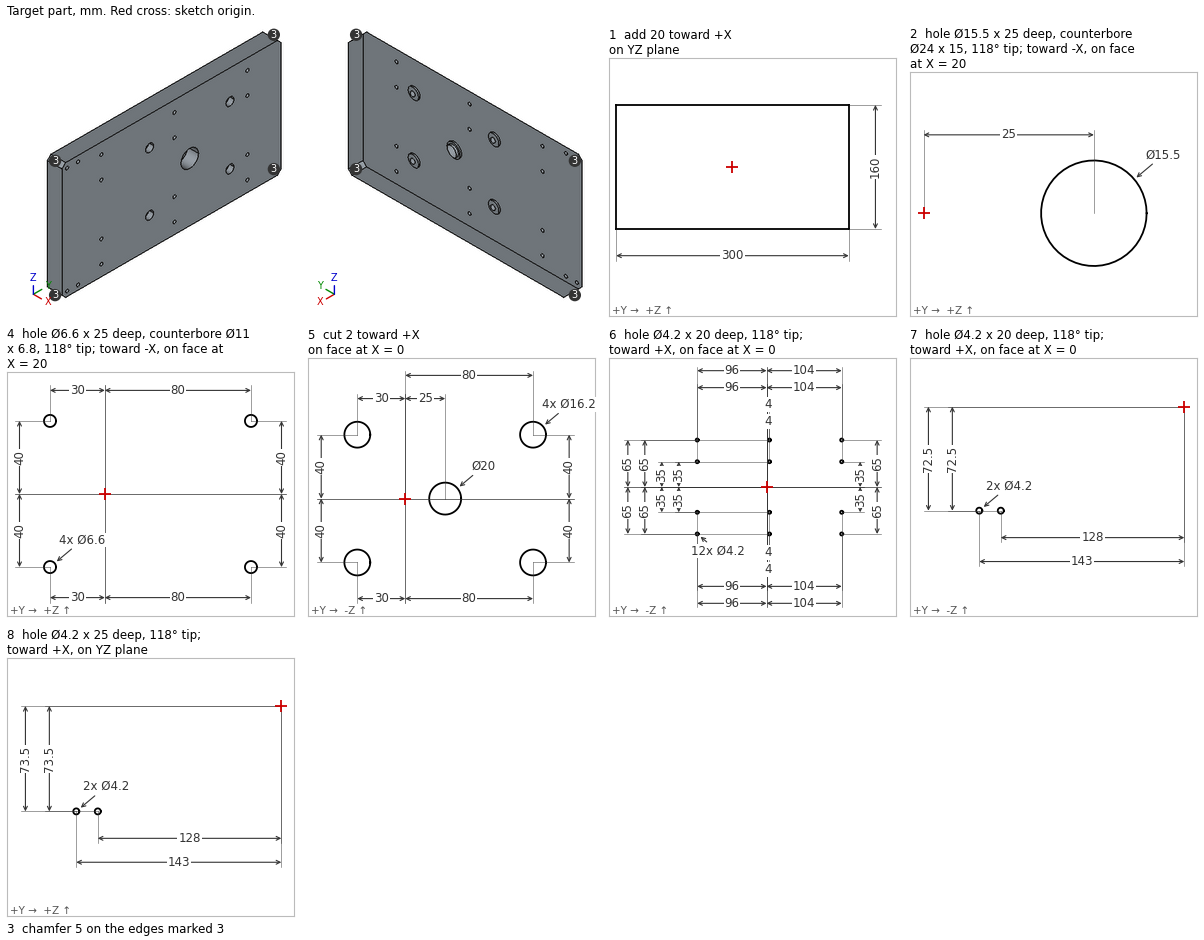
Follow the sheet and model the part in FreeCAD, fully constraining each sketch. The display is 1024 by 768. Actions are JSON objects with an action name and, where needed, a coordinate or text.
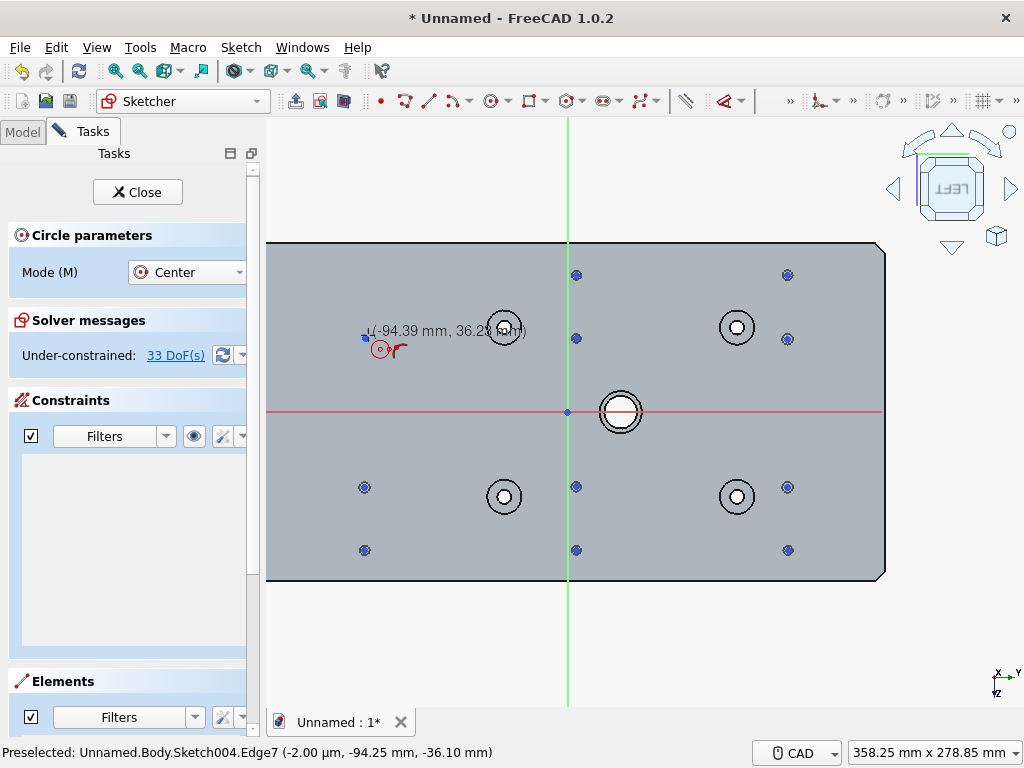
{"action": "scroll", "coordinate": [365, 275], "scroll_direction": "up", "scroll_amount": 9}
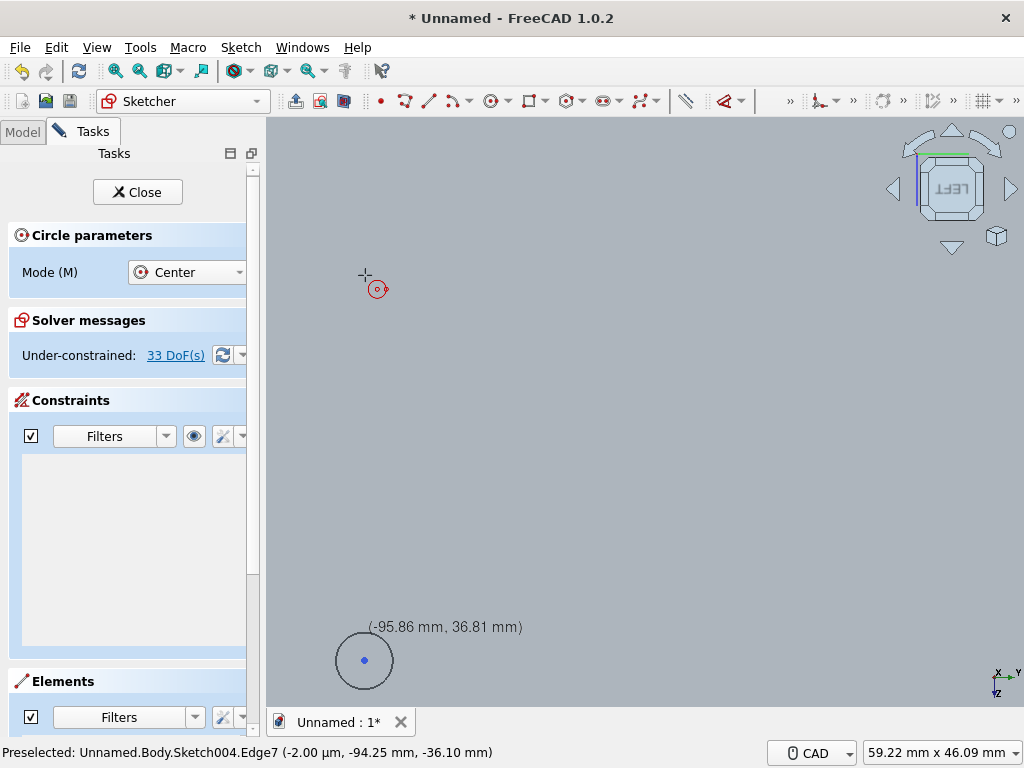
{"action": "scroll", "coordinate": [365, 275], "scroll_direction": "down", "scroll_amount": 9}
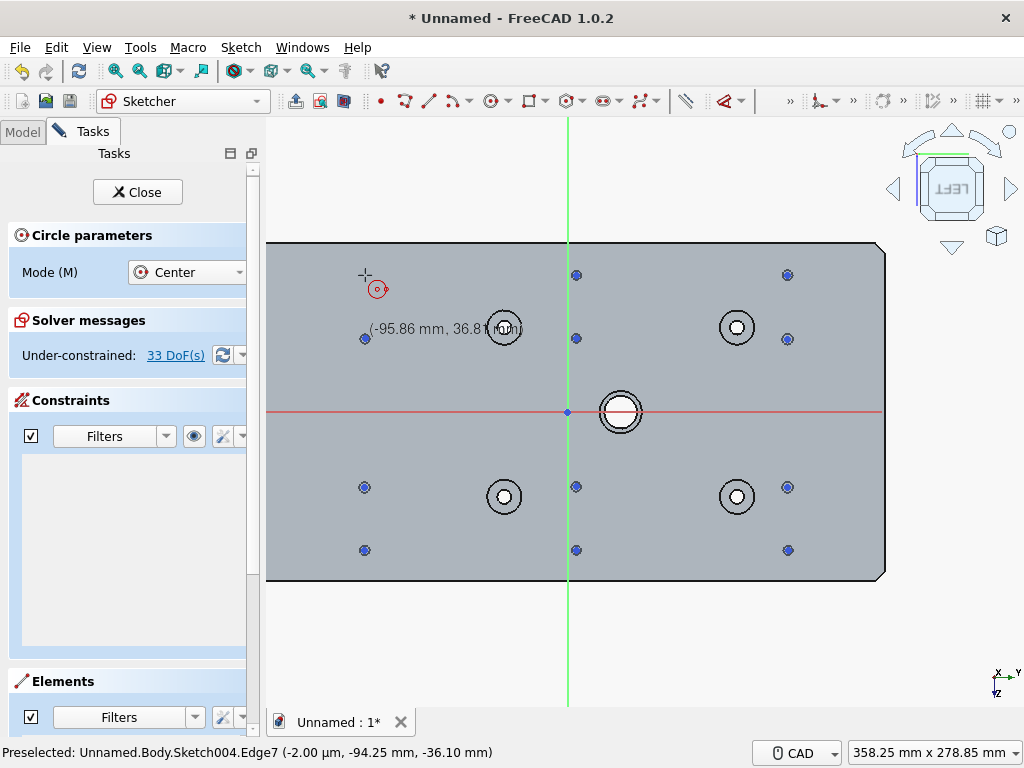
{"action": "left_click", "coordinate": [365, 275]}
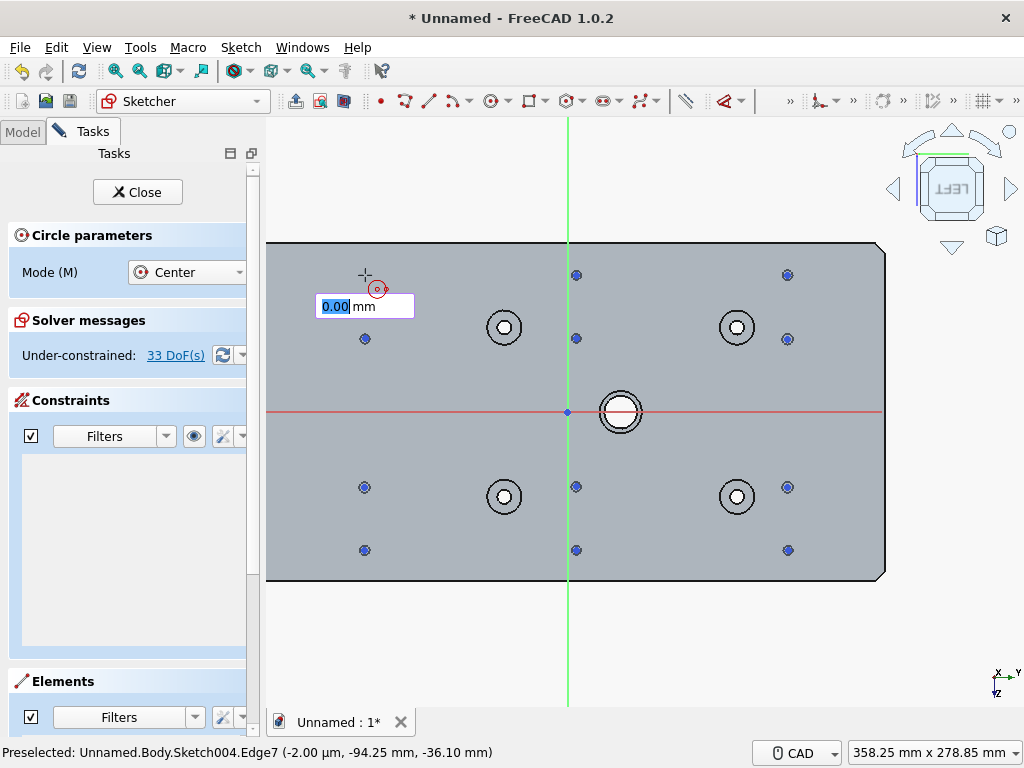
{"action": "scroll", "coordinate": [368, 272], "scroll_direction": "up", "scroll_amount": 7}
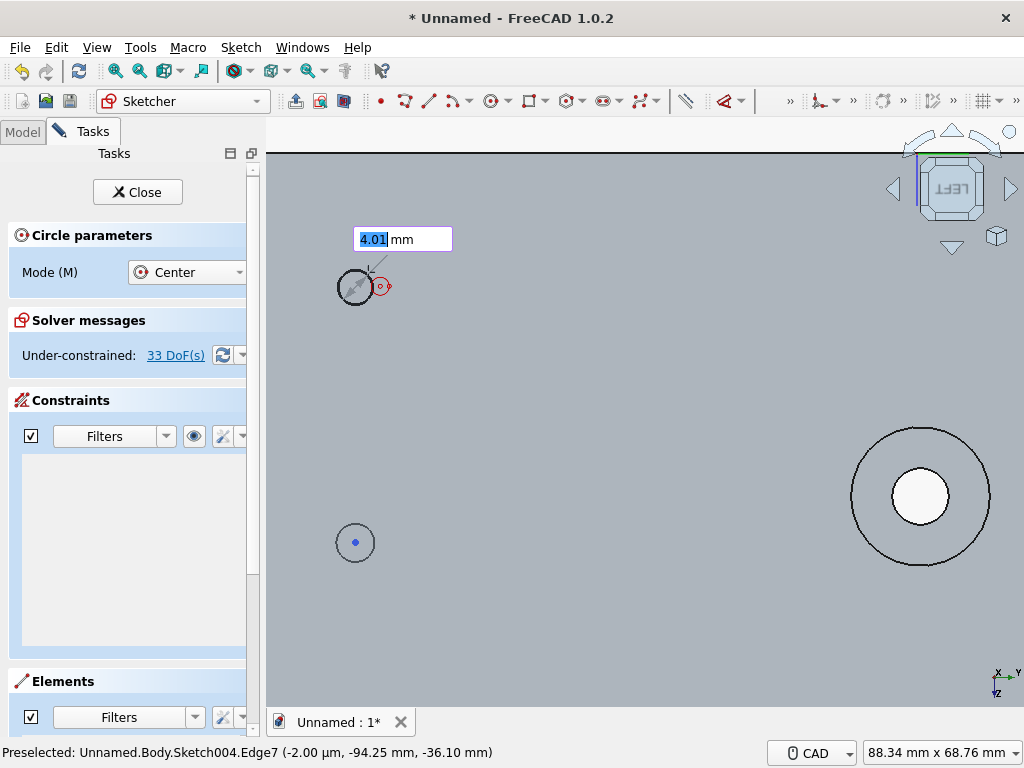
{"action": "left_click", "coordinate": [367, 269]}
{"action": "key", "text": "Escape"}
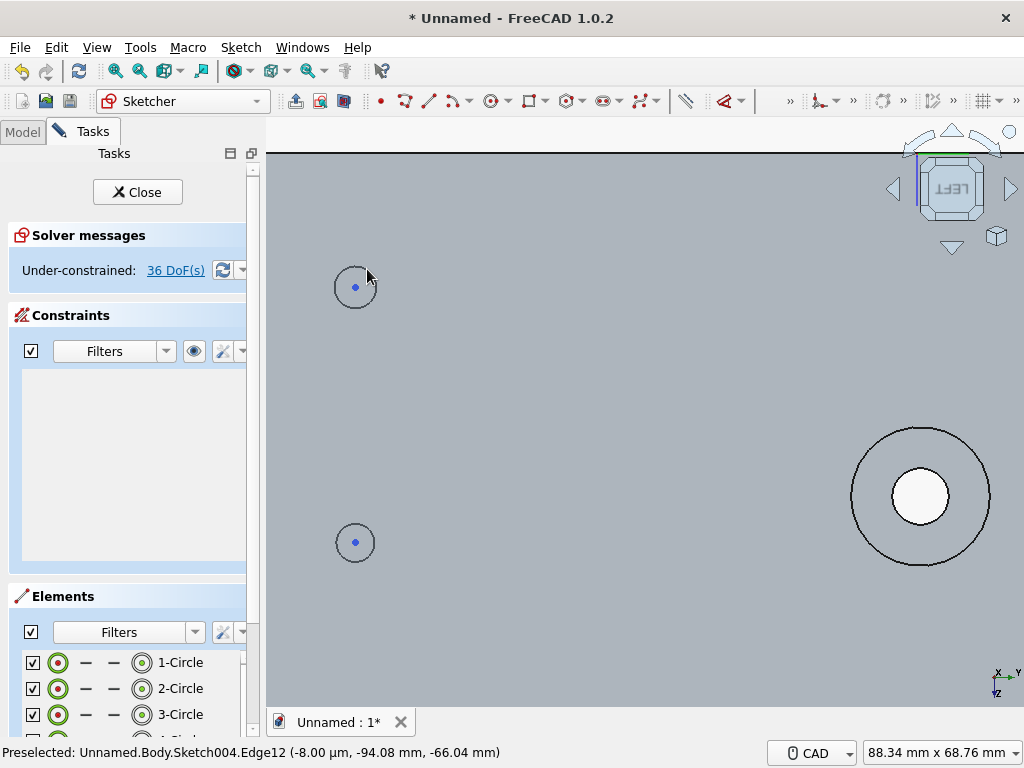
{"action": "scroll", "coordinate": [368, 272], "scroll_direction": "down", "scroll_amount": 7}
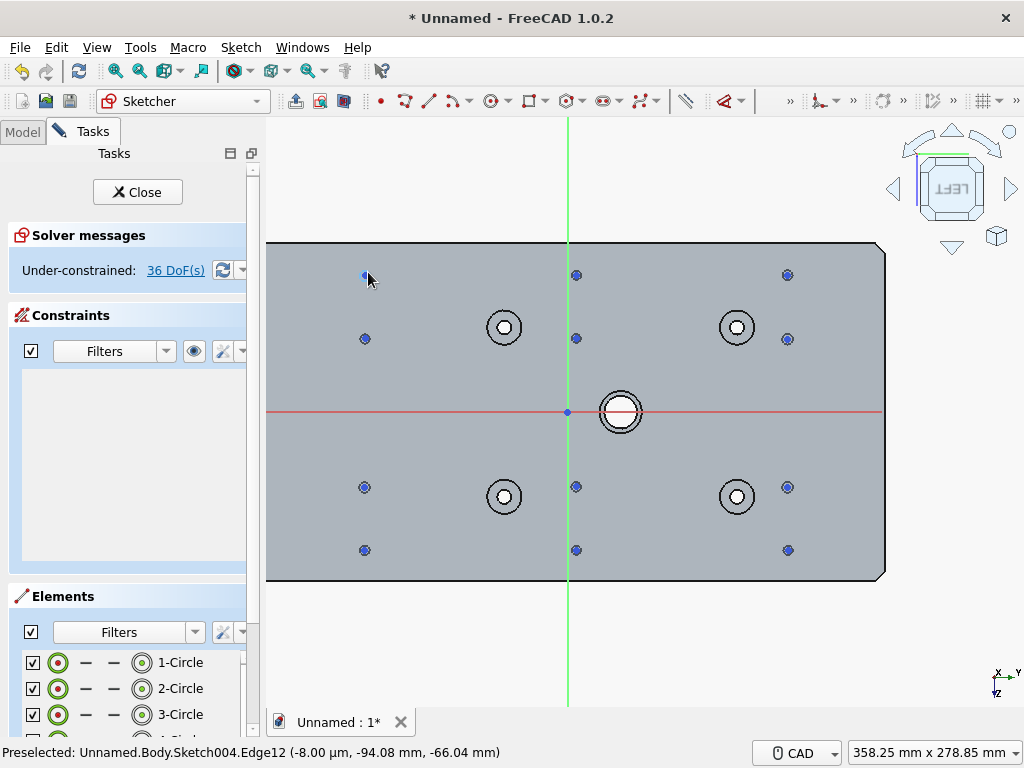
{"action": "scroll", "coordinate": [368, 547], "scroll_direction": "up", "scroll_amount": 6}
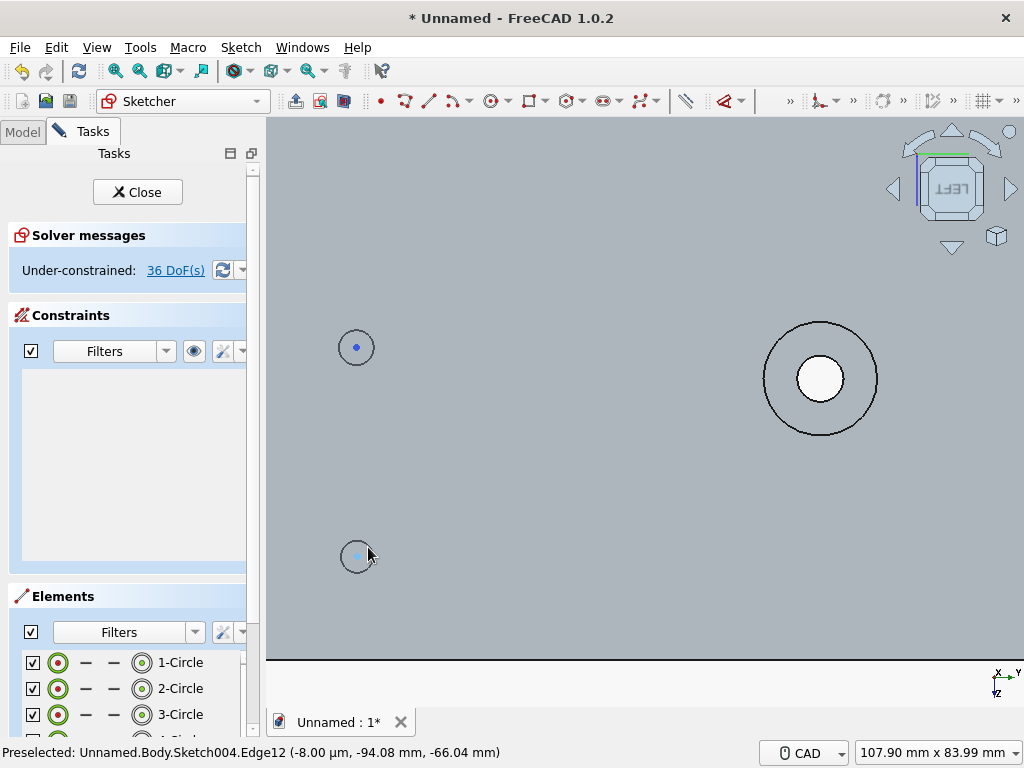
{"action": "left_click", "coordinate": [368, 545]}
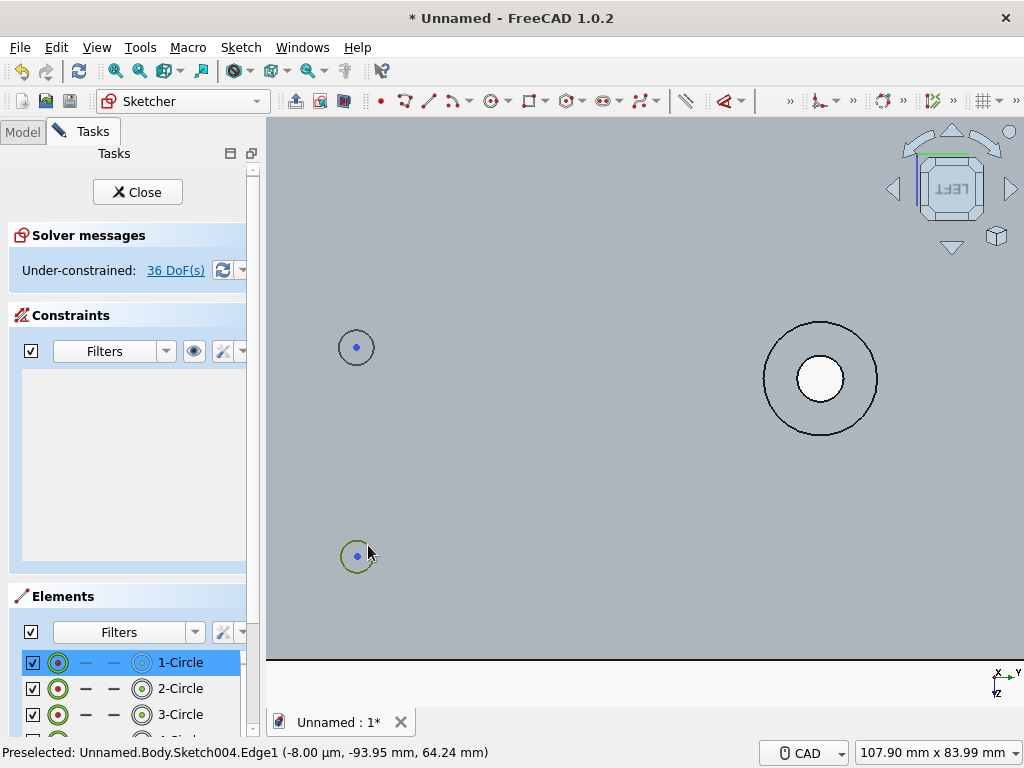
{"action": "left_click", "coordinate": [369, 335]}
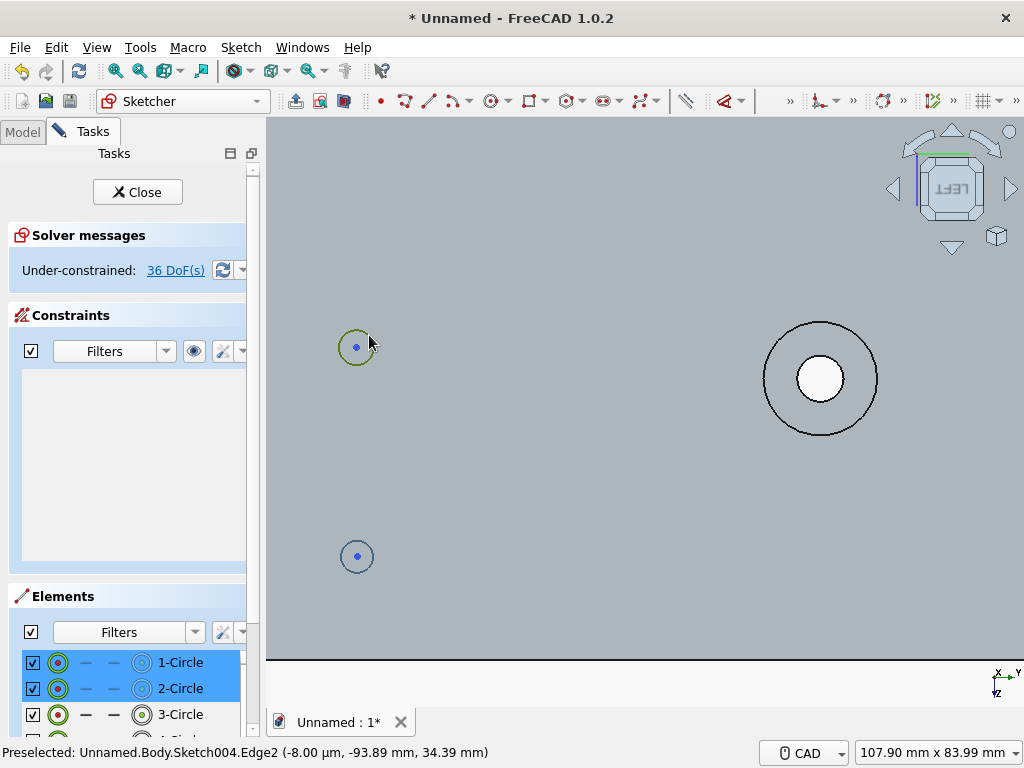
{"action": "scroll", "coordinate": [368, 547], "scroll_direction": "down", "scroll_amount": 6}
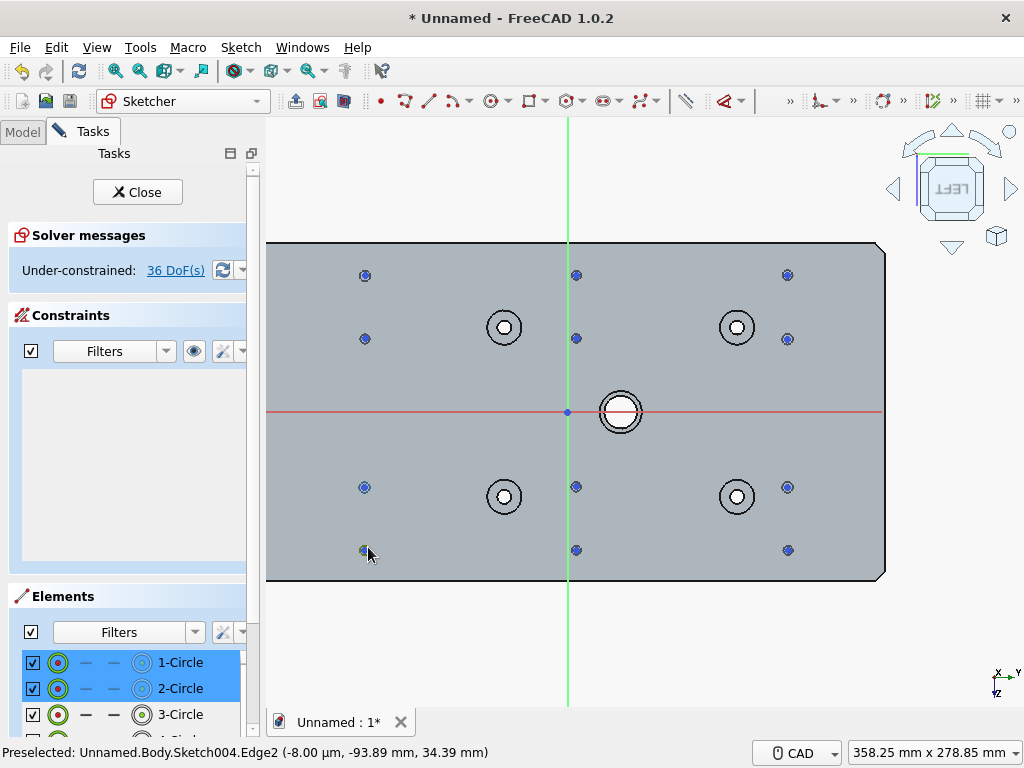
{"action": "scroll", "coordinate": [580, 547], "scroll_direction": "up", "scroll_amount": 6}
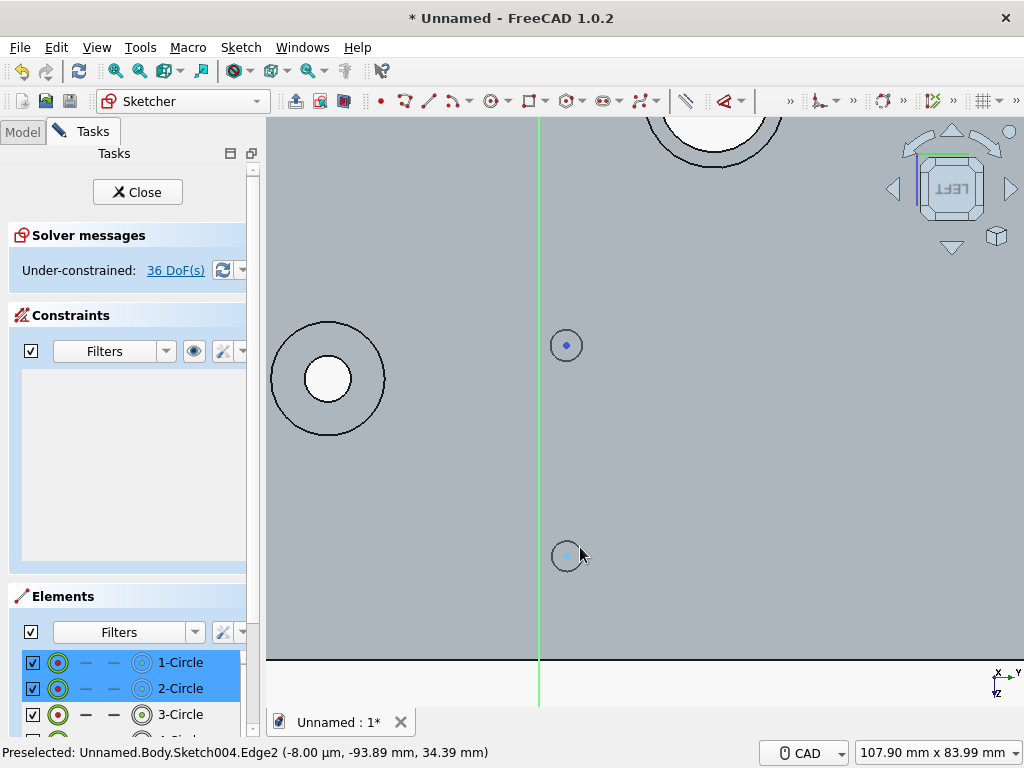
{"action": "left_click", "coordinate": [578, 546]}